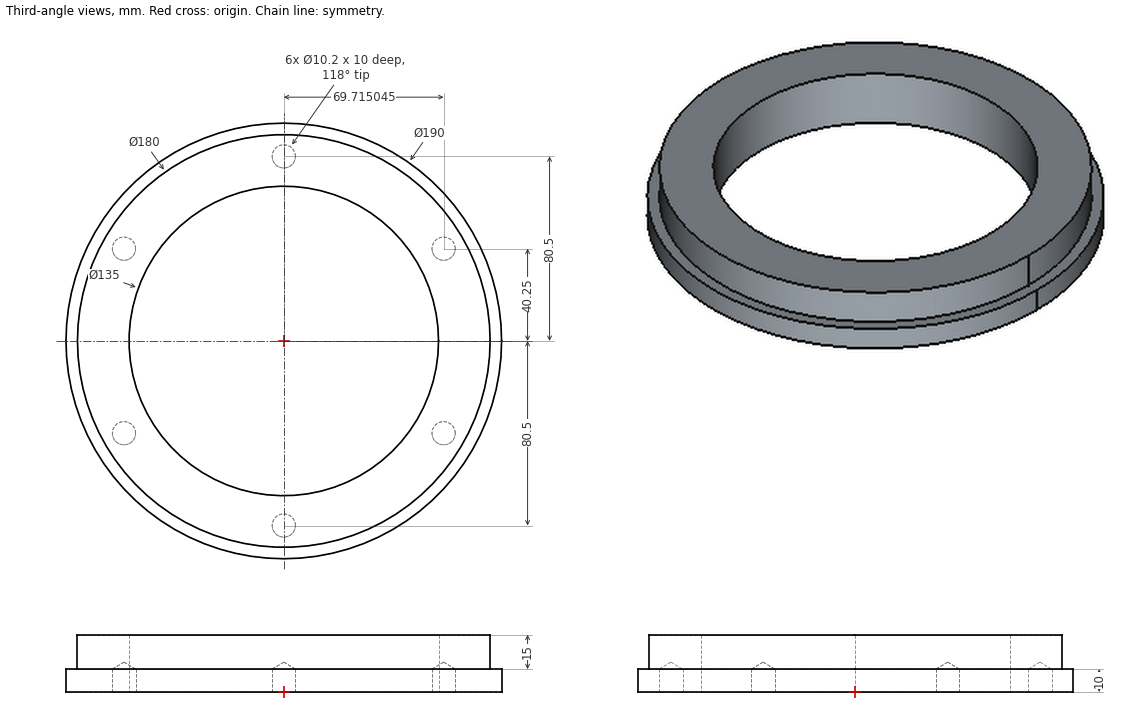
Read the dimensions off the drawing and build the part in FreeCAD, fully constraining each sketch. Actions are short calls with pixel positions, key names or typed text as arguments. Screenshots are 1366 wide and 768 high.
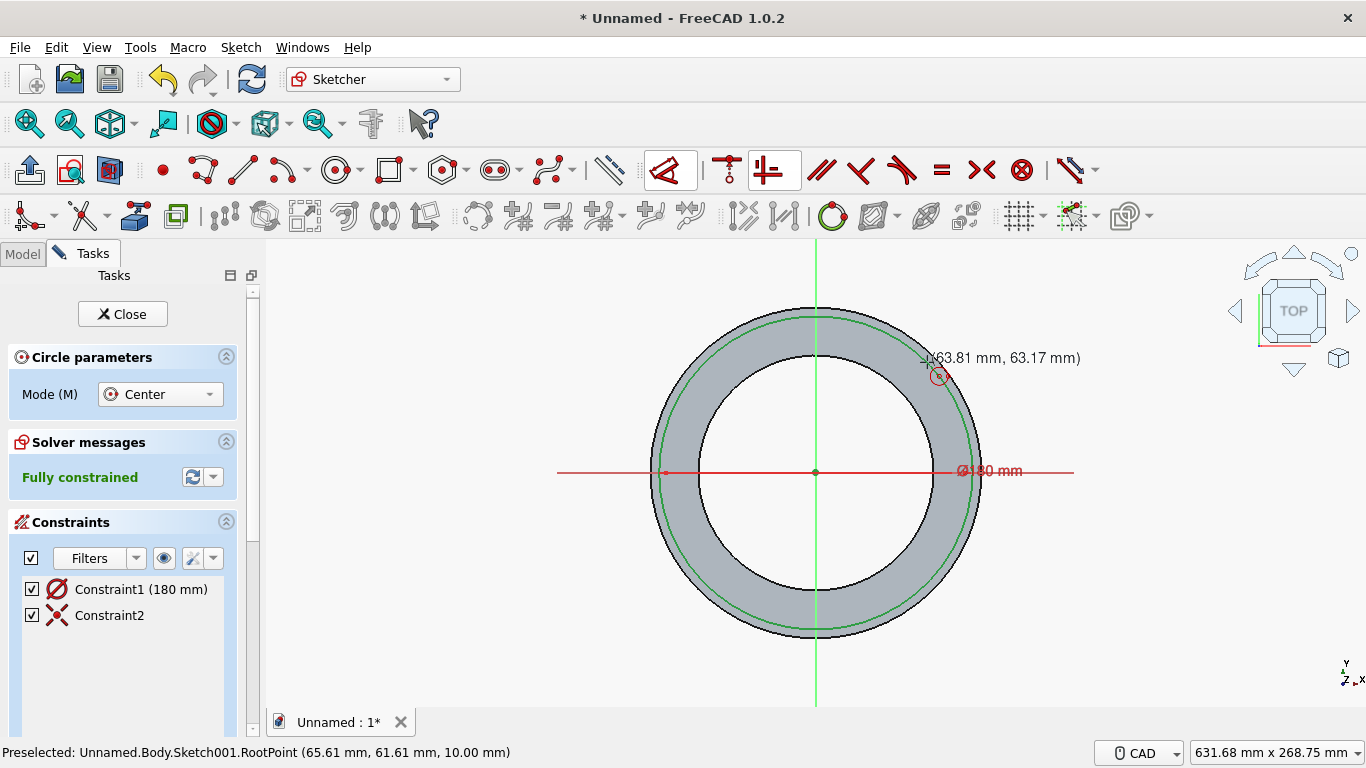
click(816, 473)
move(899, 390)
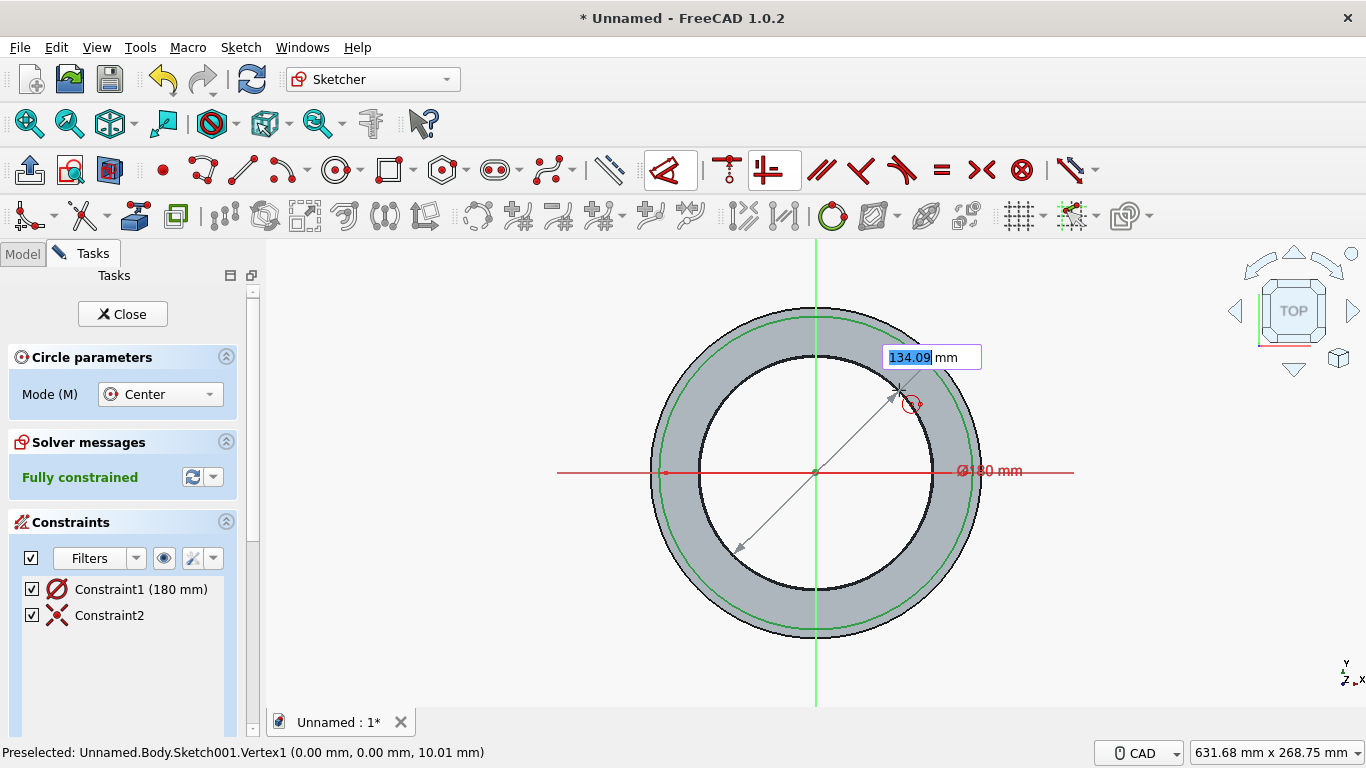
text(135)
key(Return)
key(Escape)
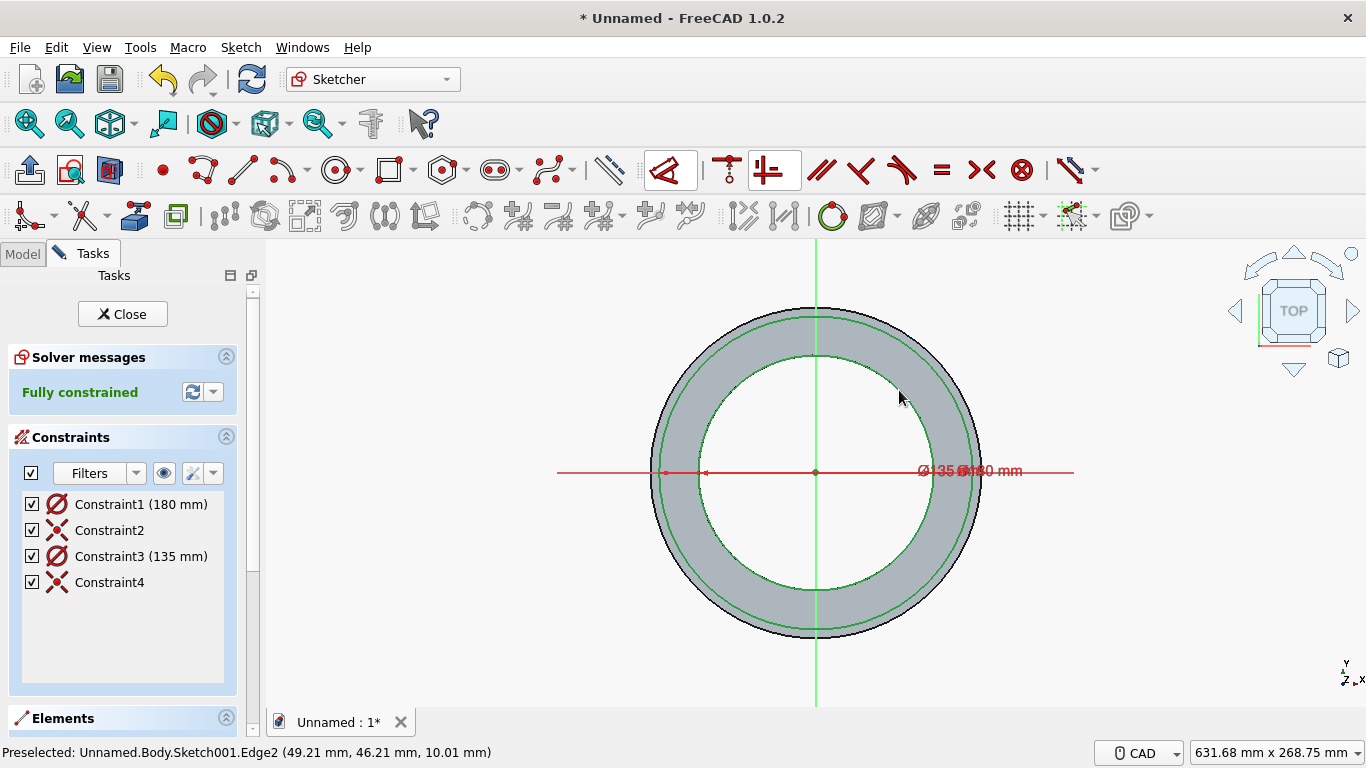
click(123, 314)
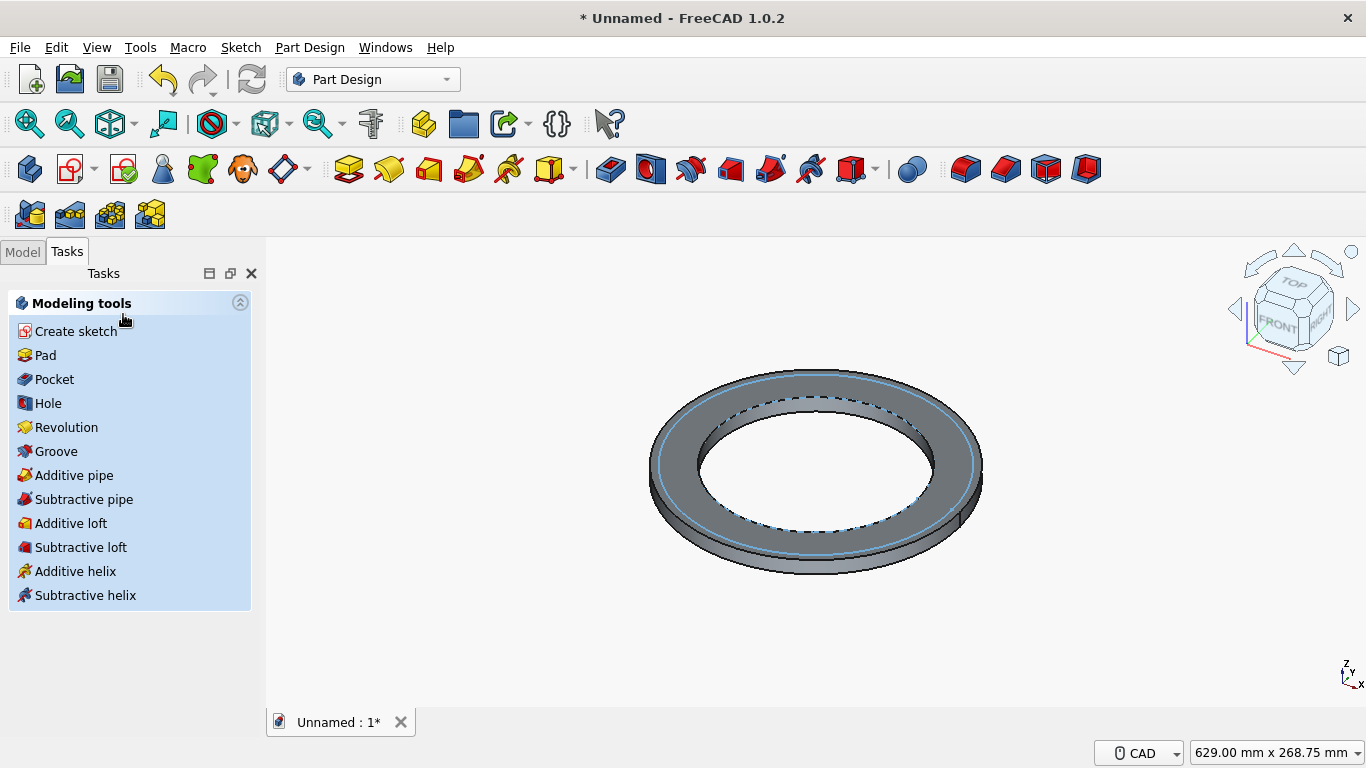
click(350, 170)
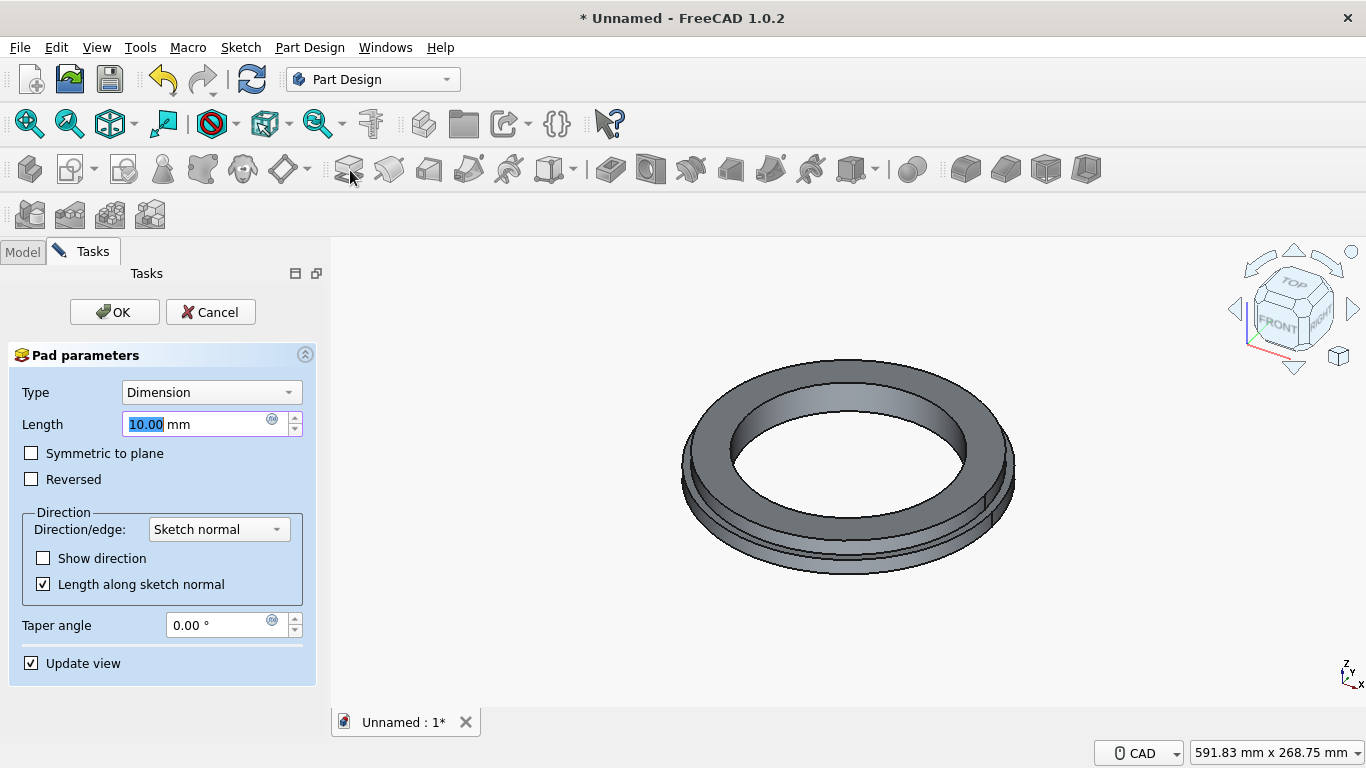
text(15)
key(Tab)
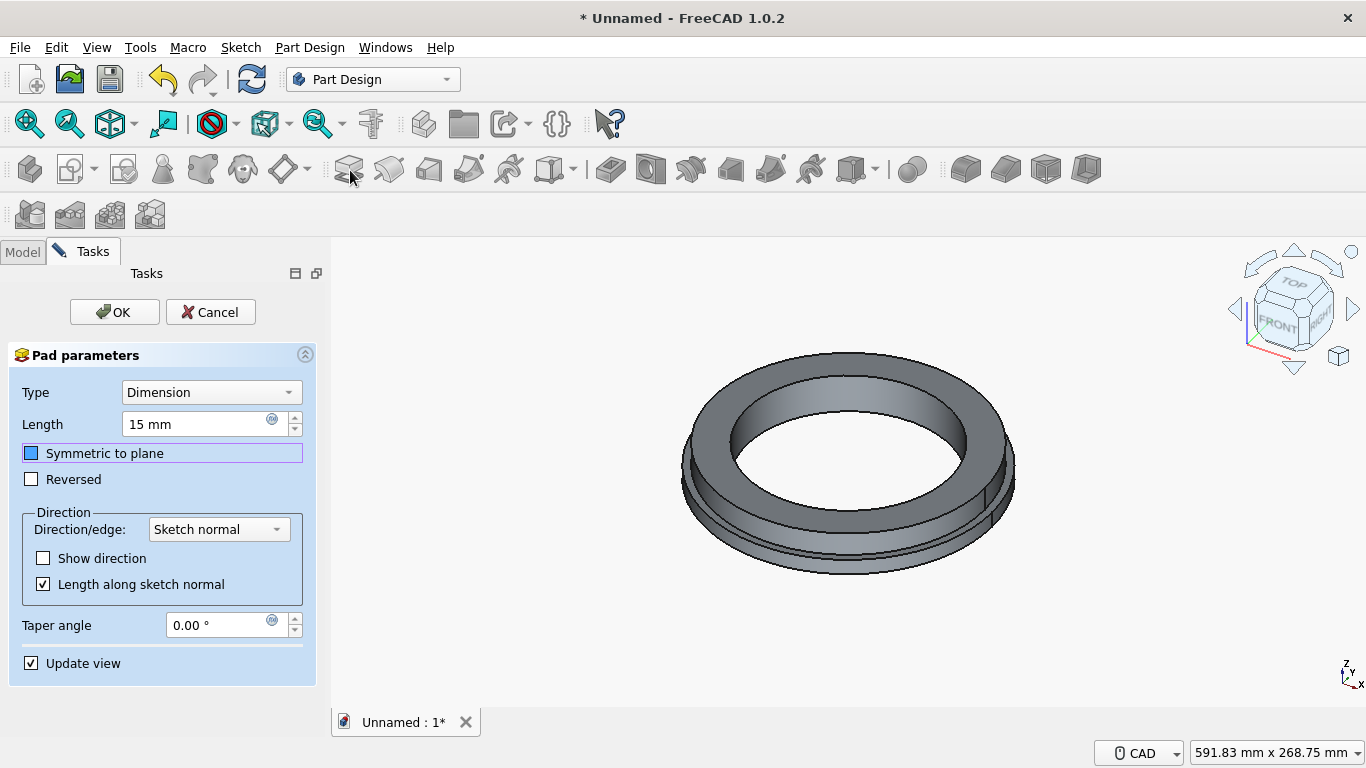
click(115, 312)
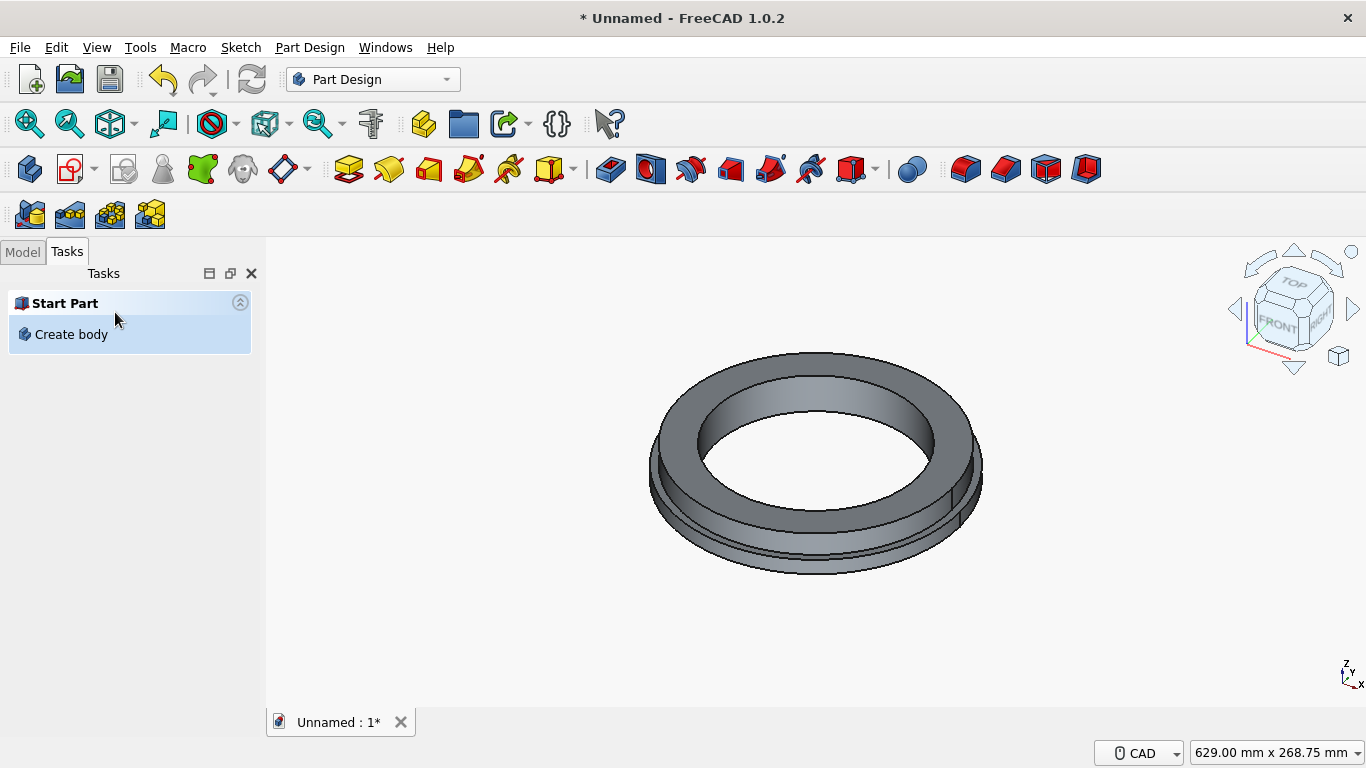
key(5)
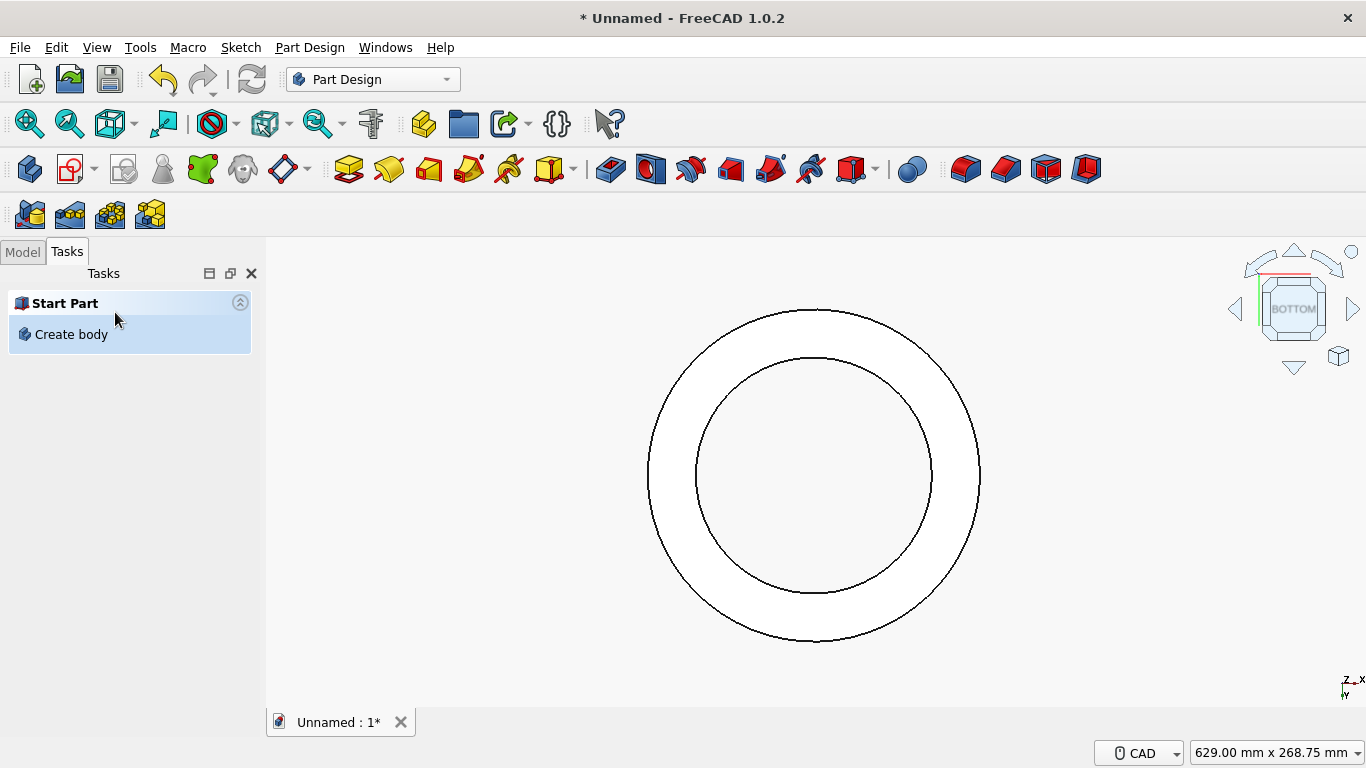
click(956, 475)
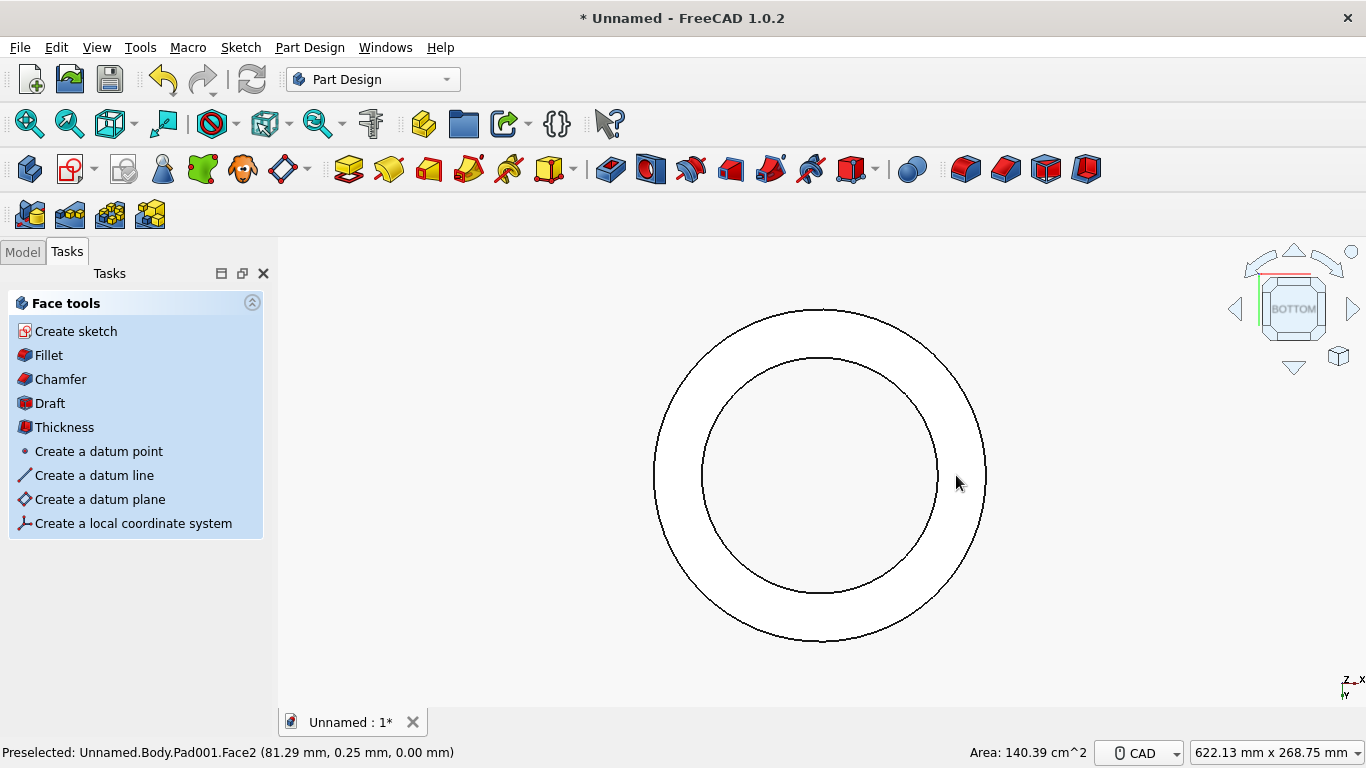
click(70, 170)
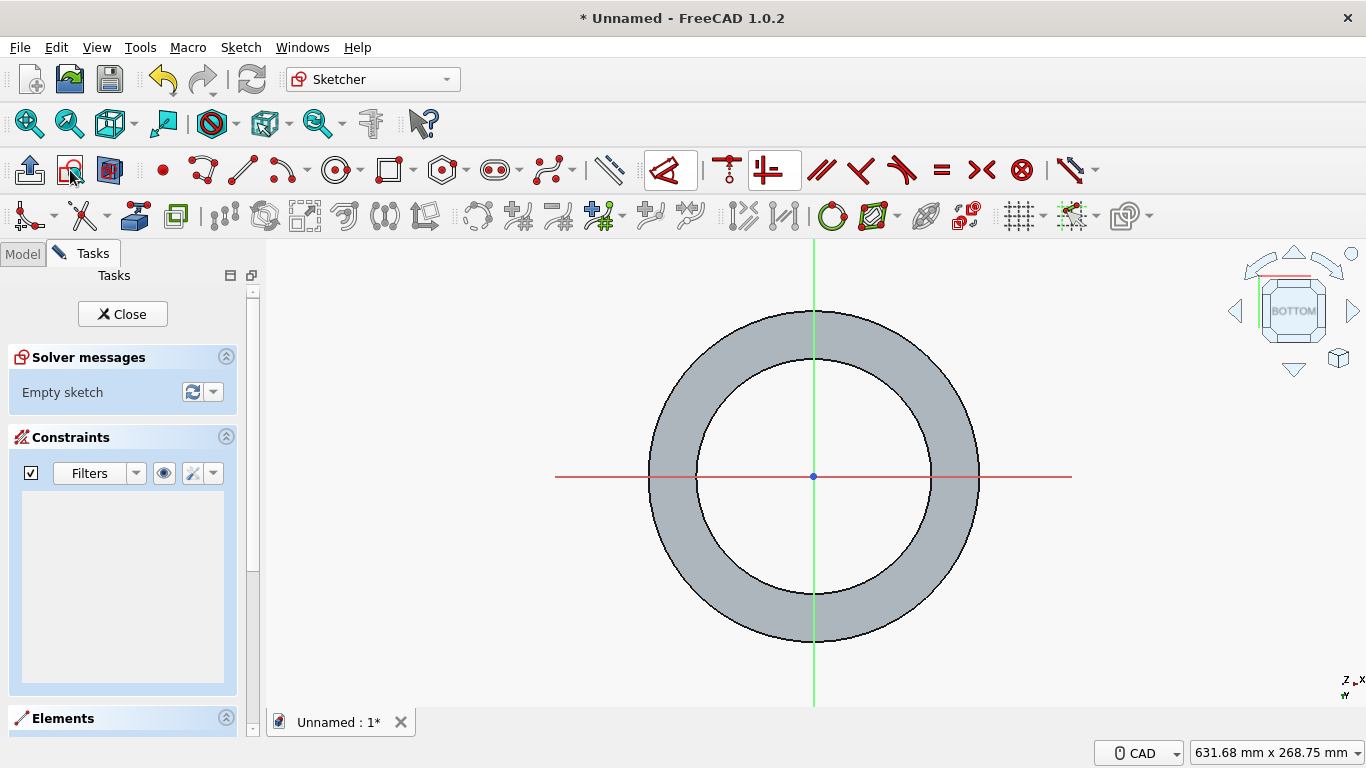
key(g)
key(c)